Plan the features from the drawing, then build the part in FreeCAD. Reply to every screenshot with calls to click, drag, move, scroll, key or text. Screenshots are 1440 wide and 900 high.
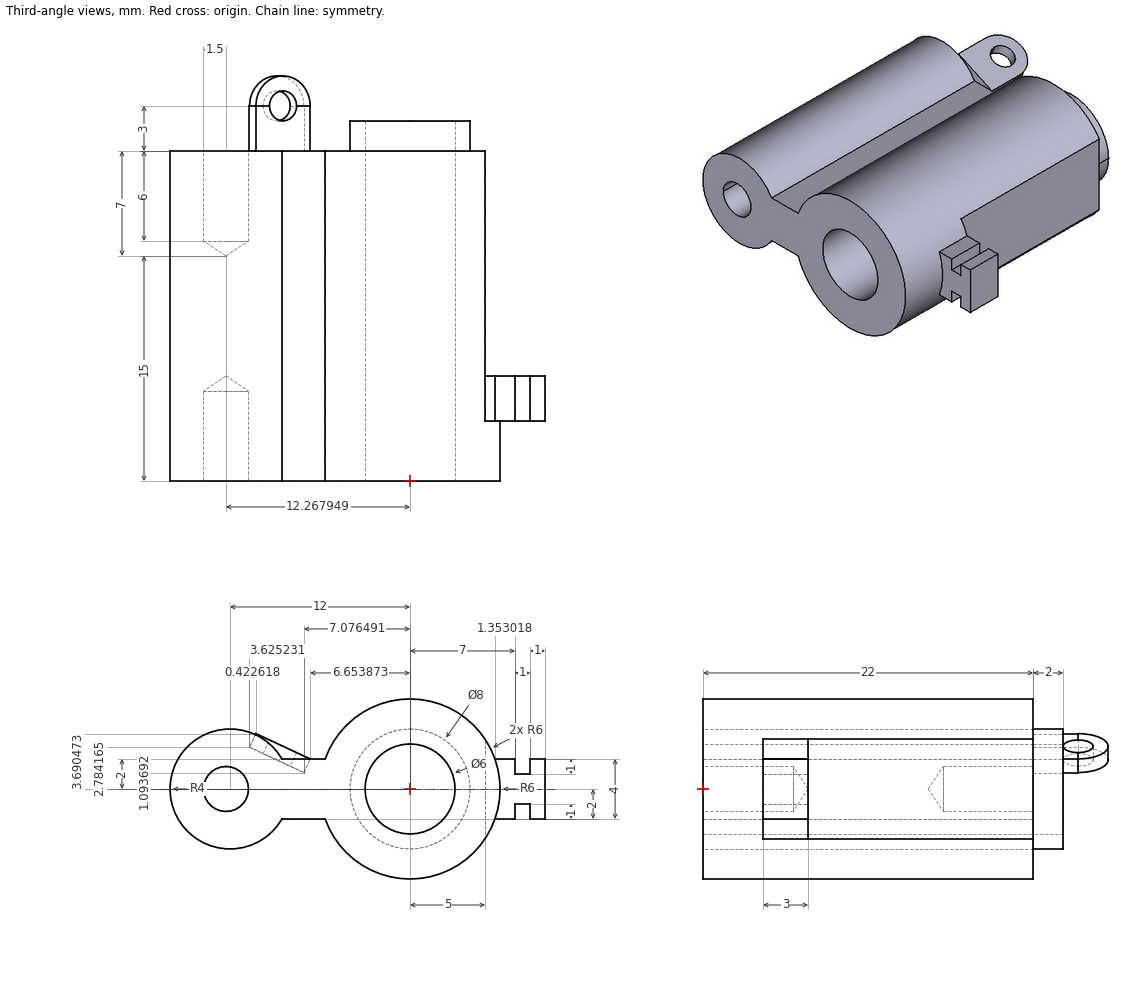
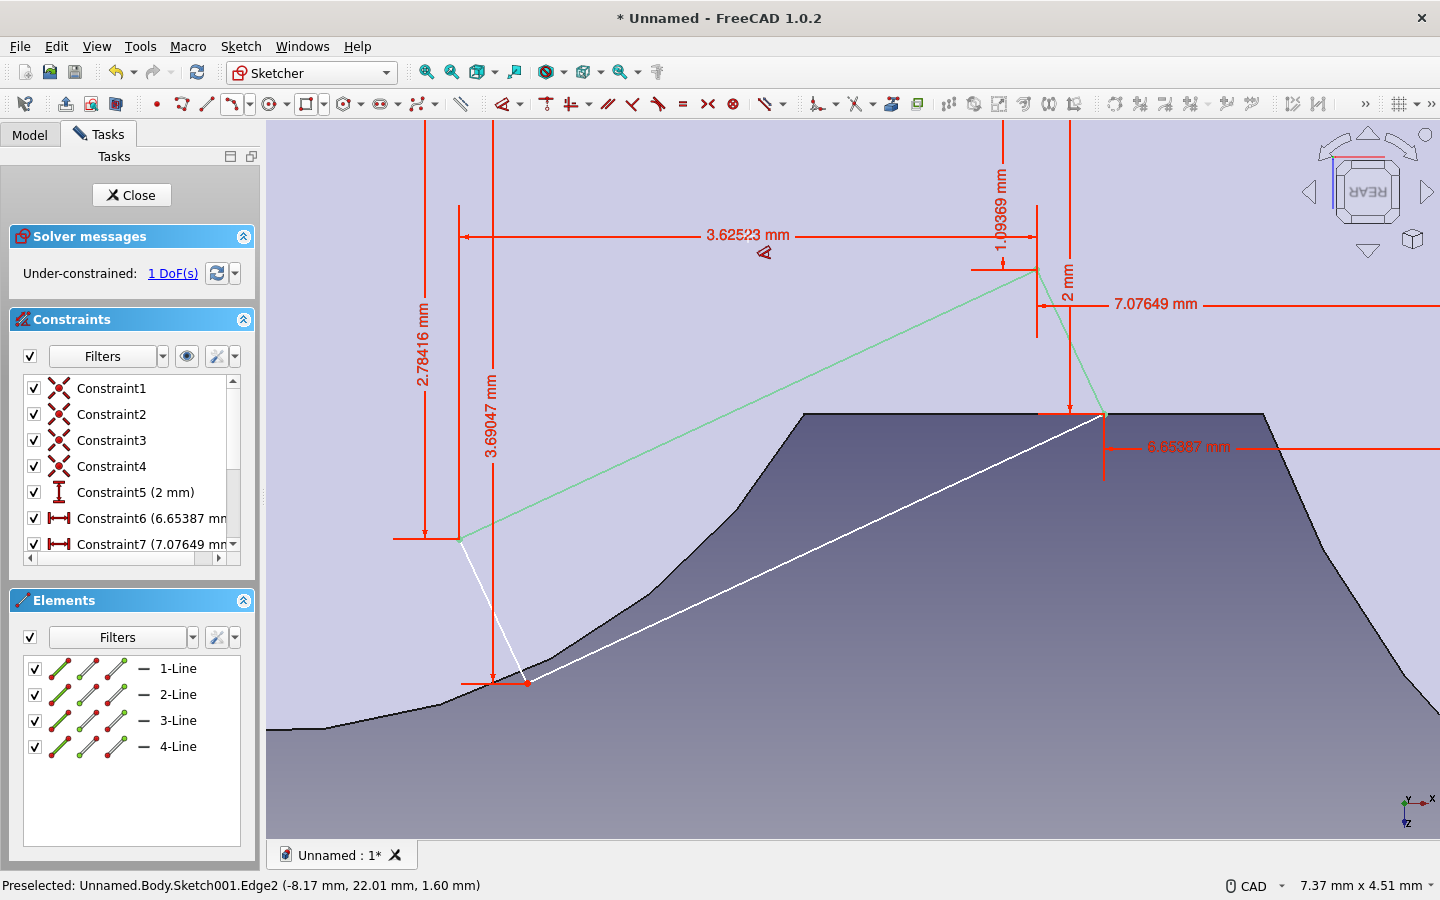
click(480, 583)
click(493, 718)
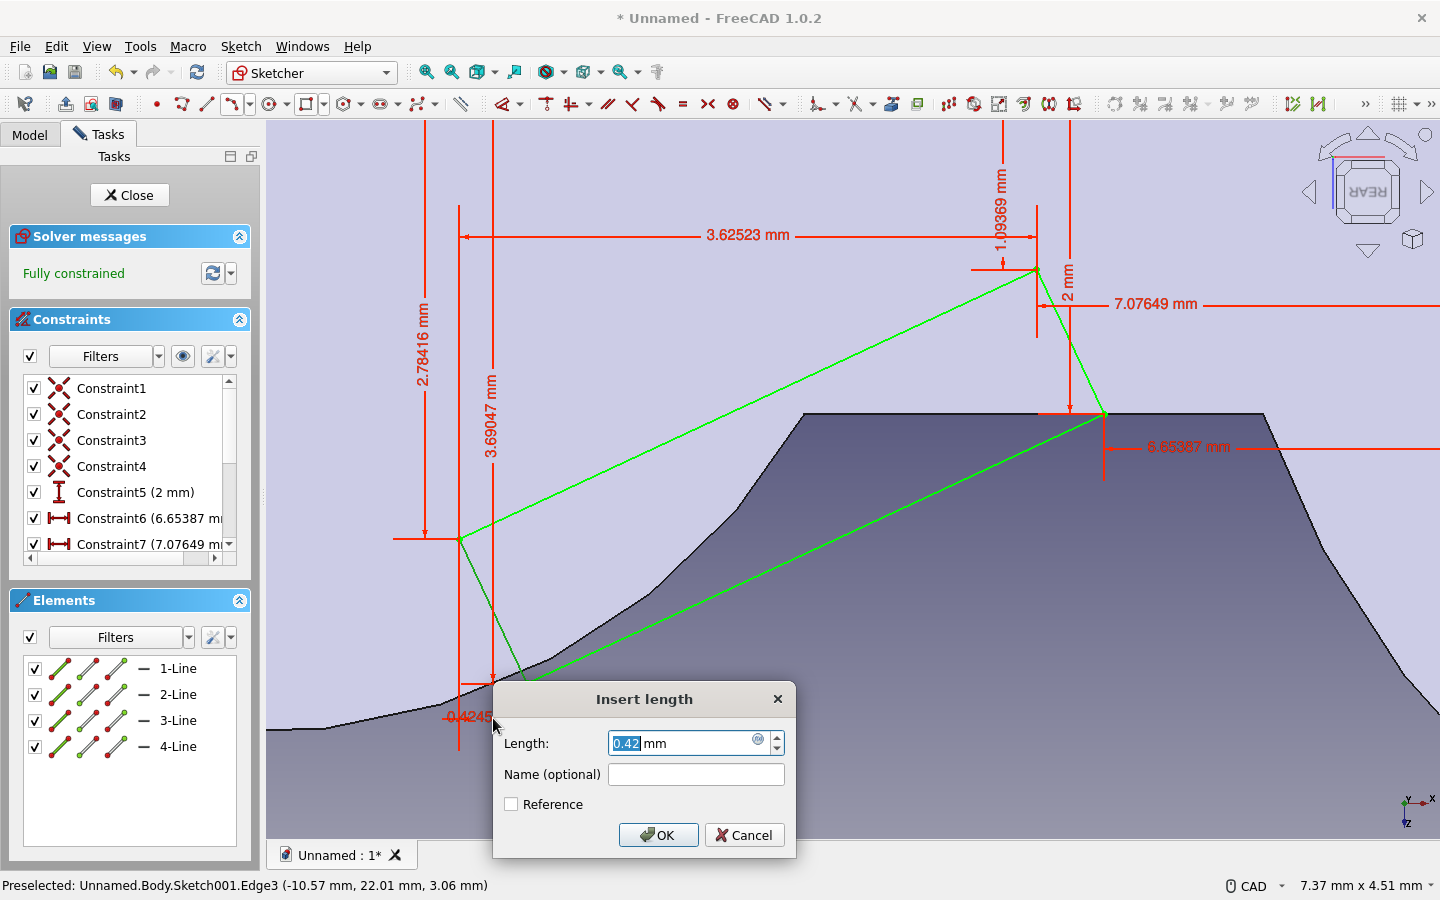
text(0.422618)
key(Return)
key(Escape)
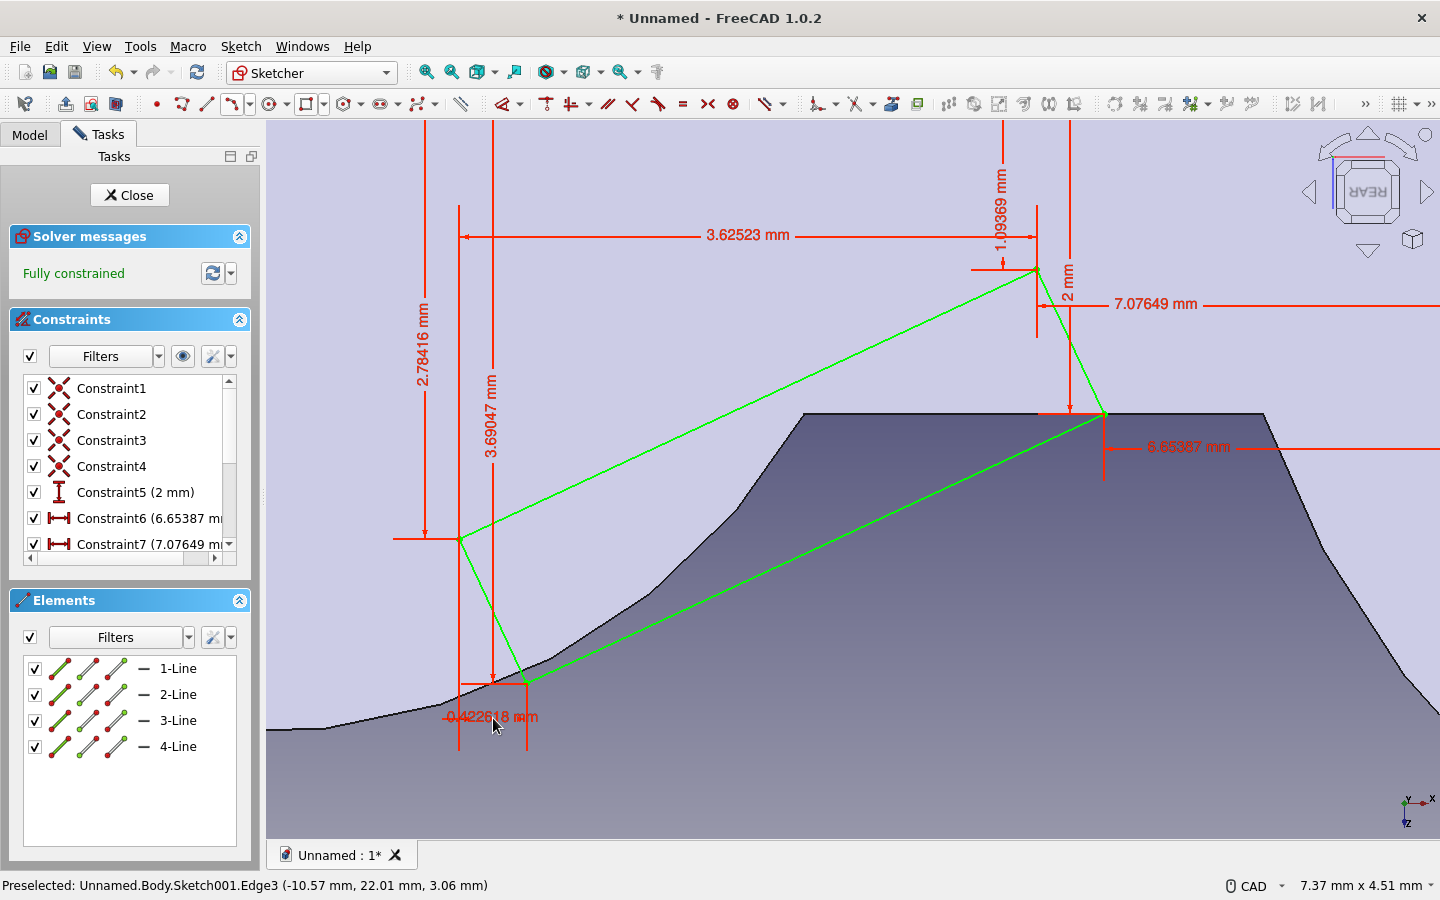
click(130, 195)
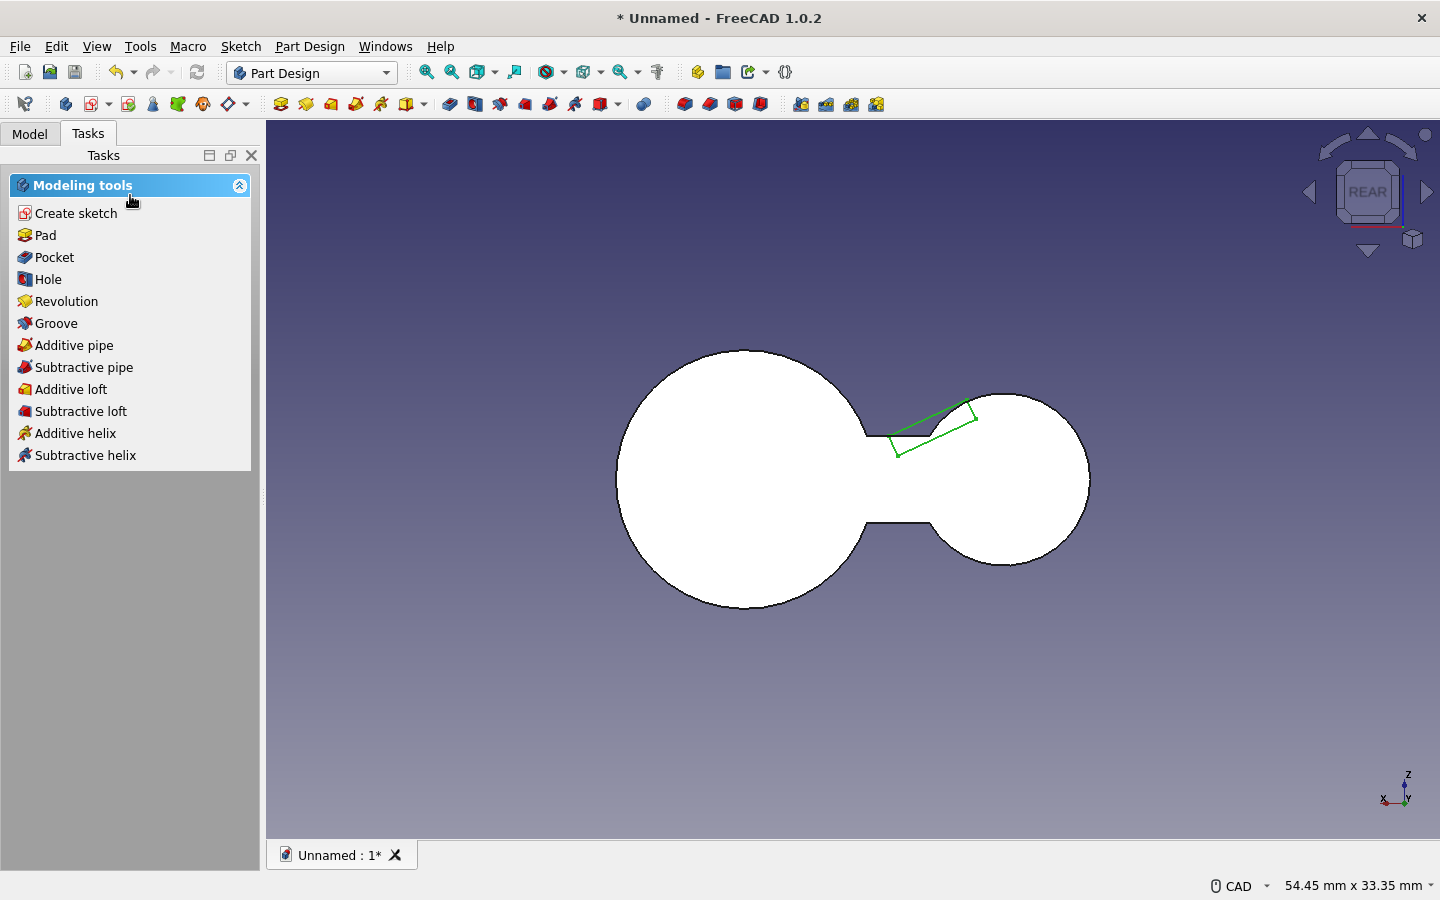
click(281, 104)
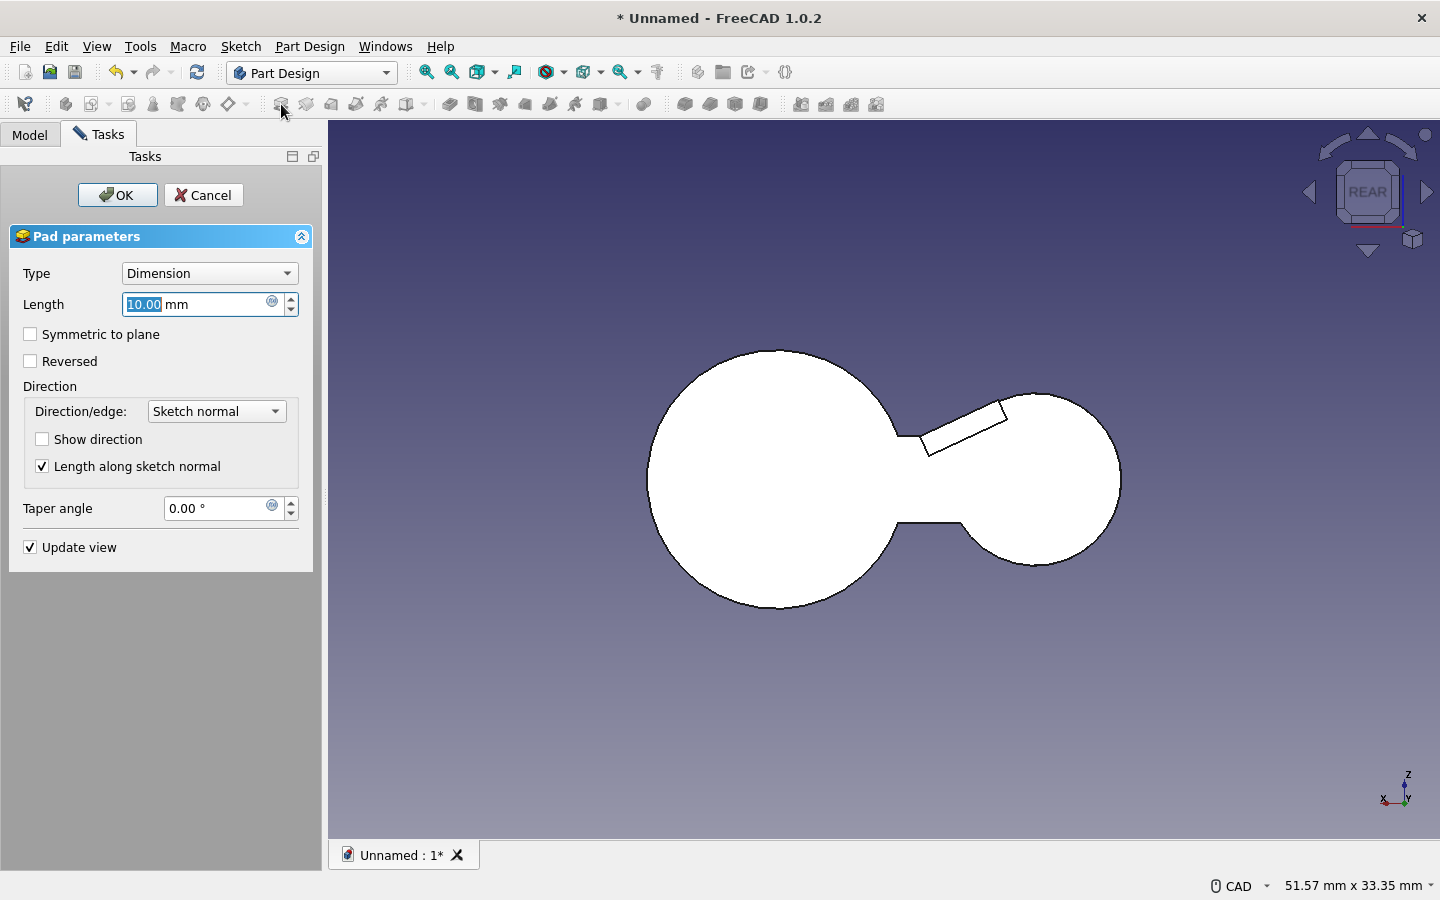
text(3)
key(Tab)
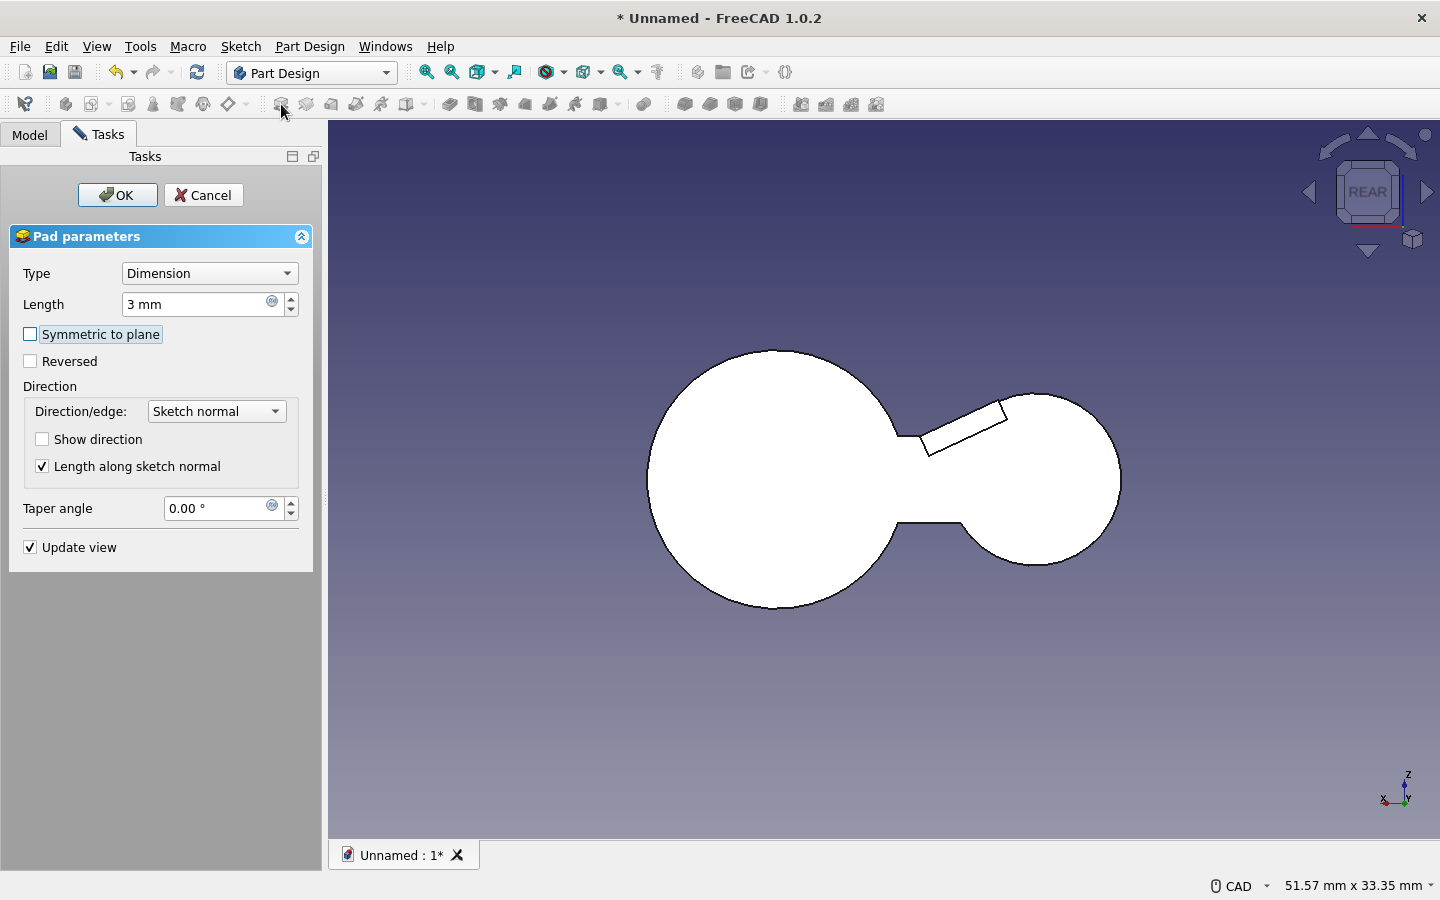
click(118, 195)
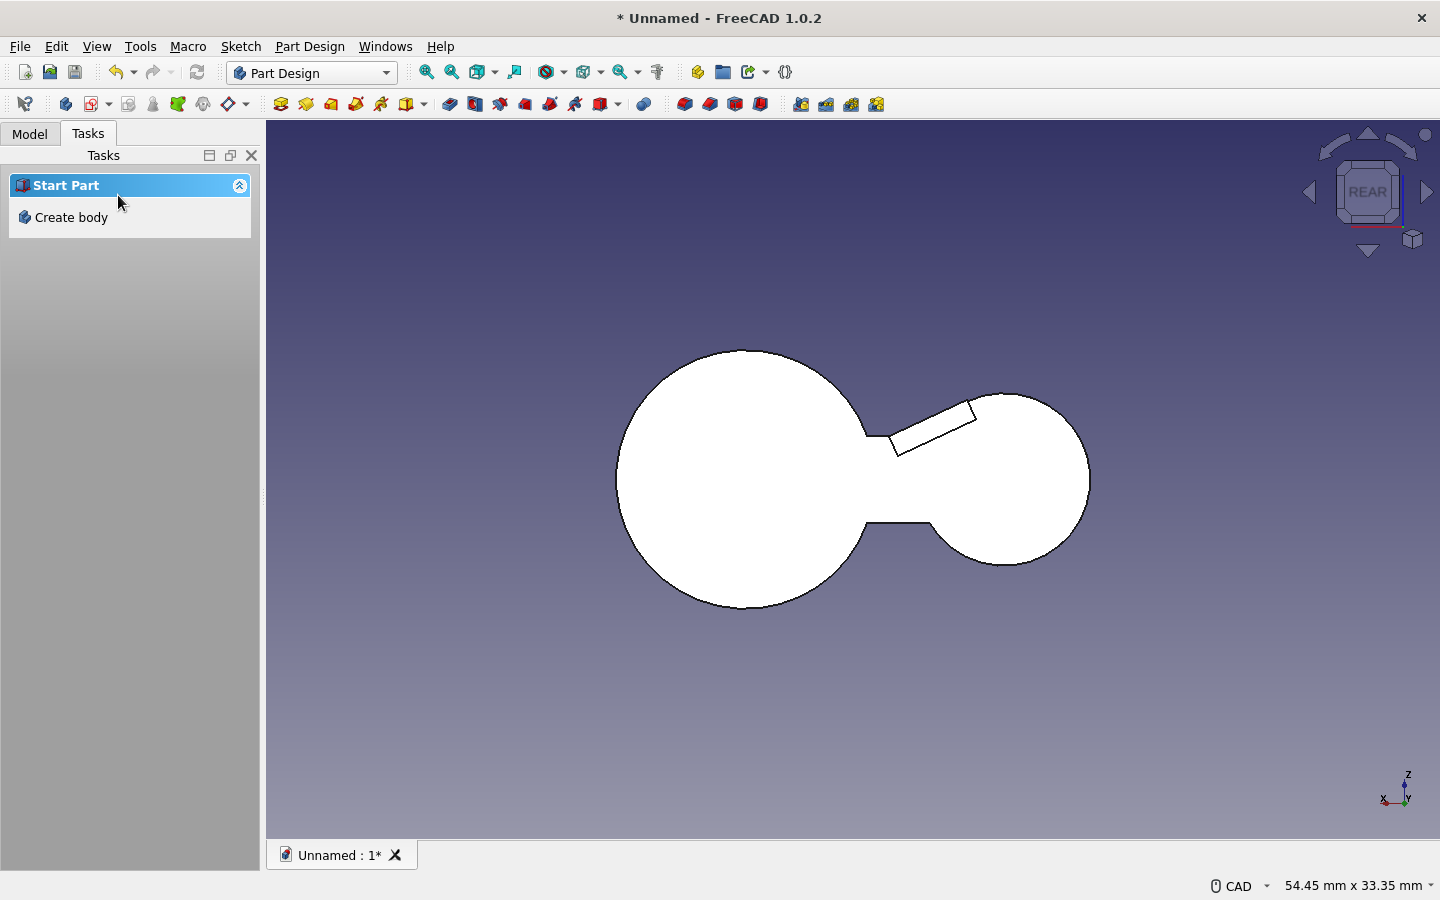
click(427, 72)